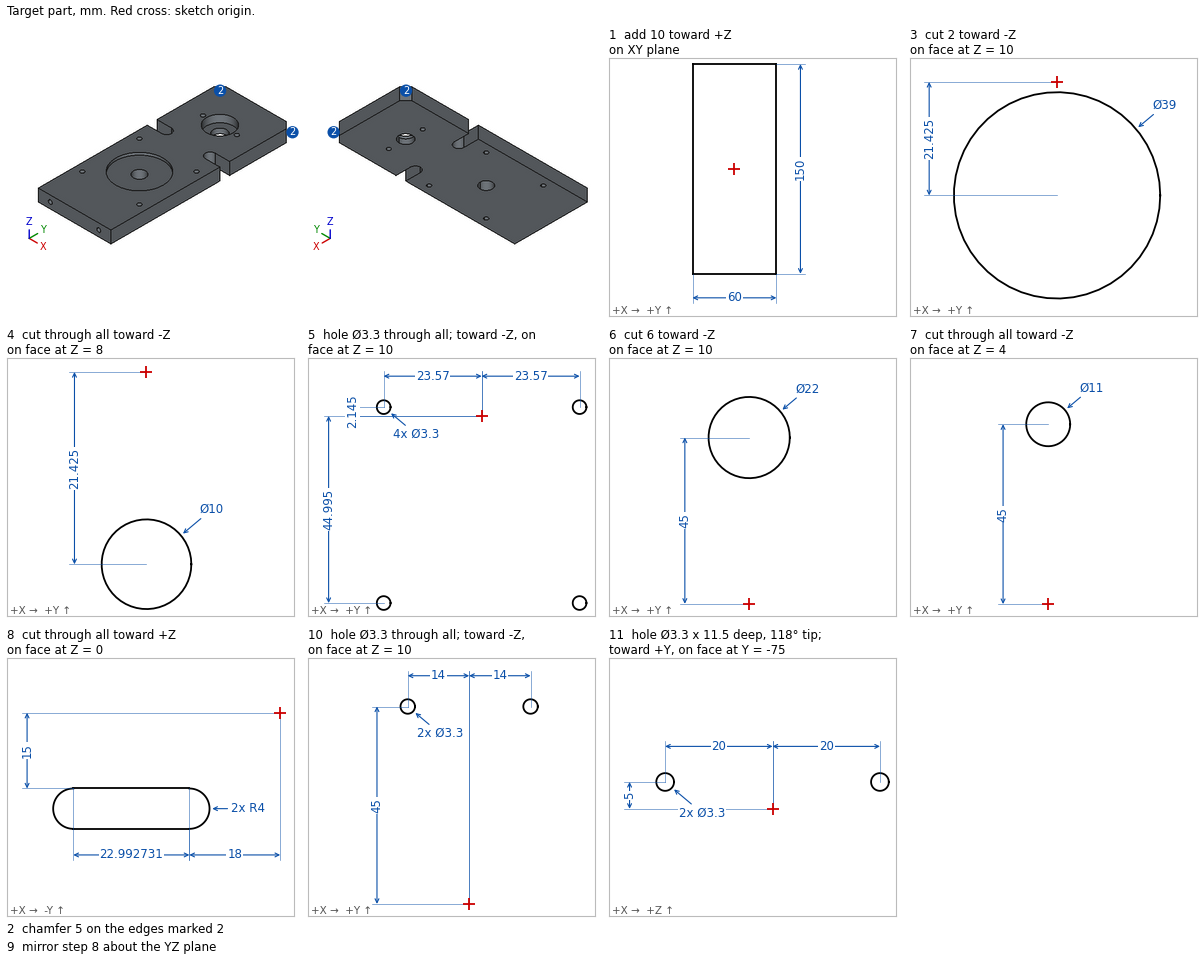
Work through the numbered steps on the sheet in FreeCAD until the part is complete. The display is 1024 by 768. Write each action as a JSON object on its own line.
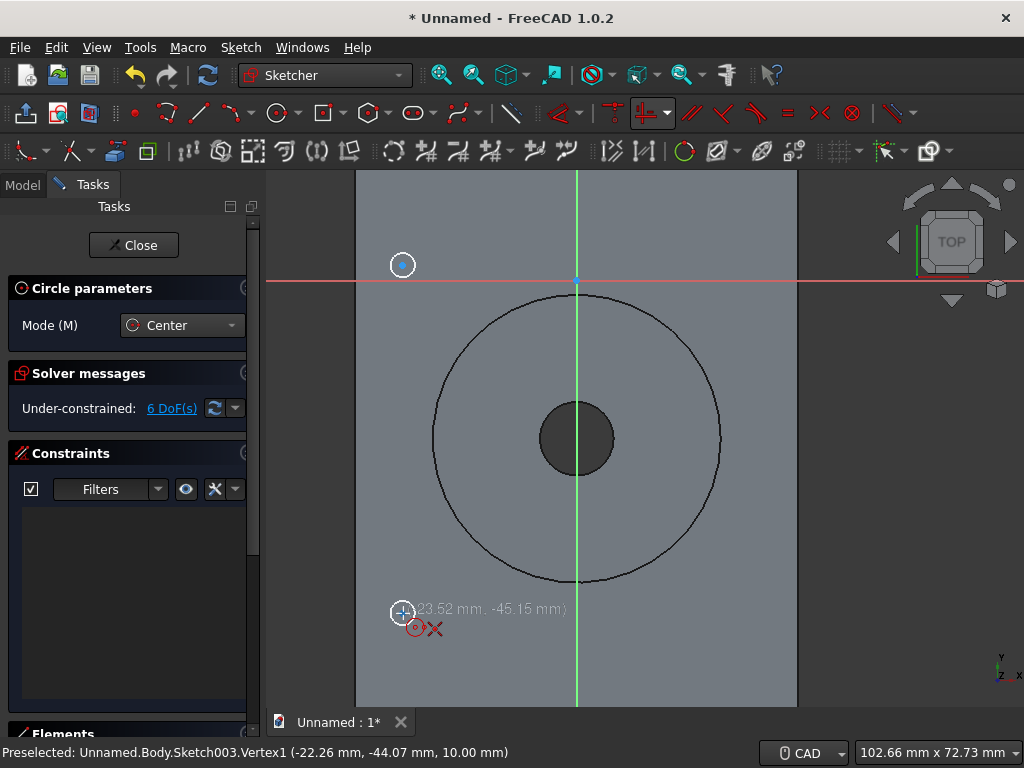
{"action": "scroll", "coordinate": [751, 265], "scroll_direction": "up", "scroll_amount": 4}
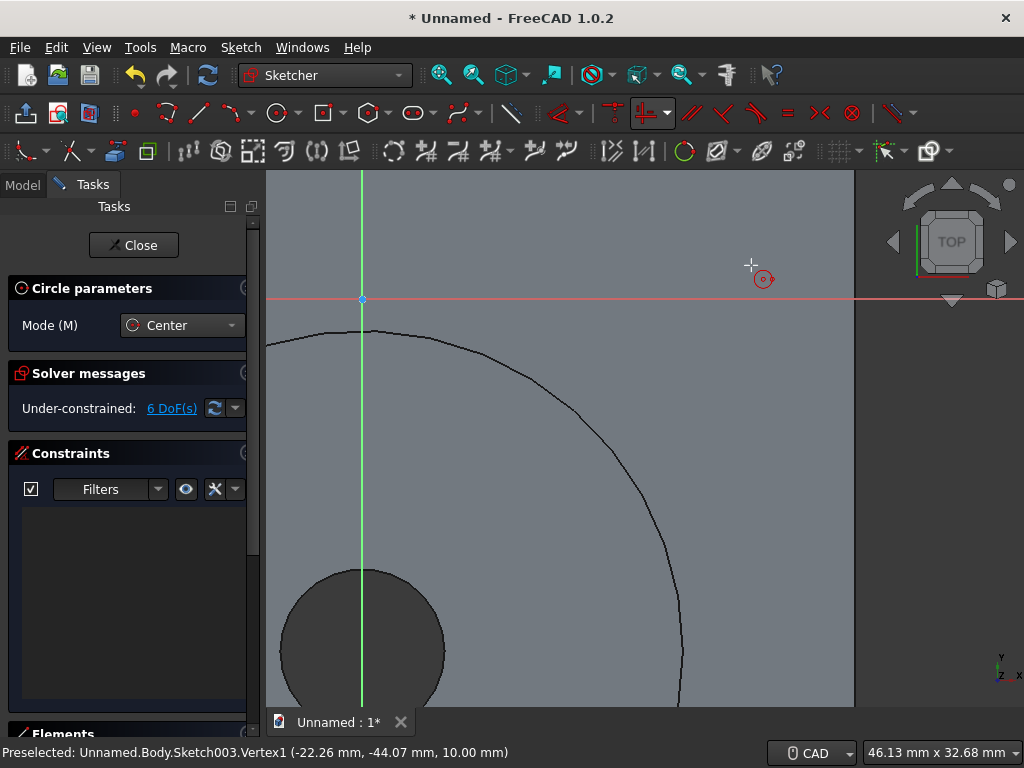
{"action": "left_click", "coordinate": [750, 264]}
{"action": "left_click", "coordinate": [769, 245]}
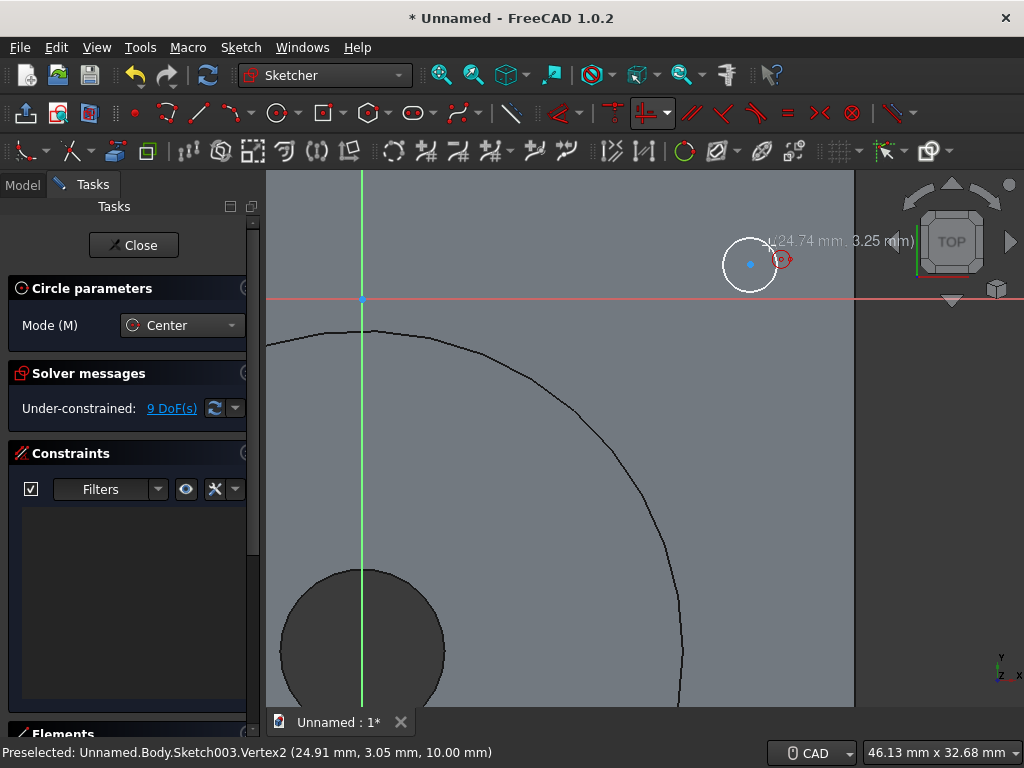
{"action": "scroll", "coordinate": [751, 265], "scroll_direction": "down", "scroll_amount": 4}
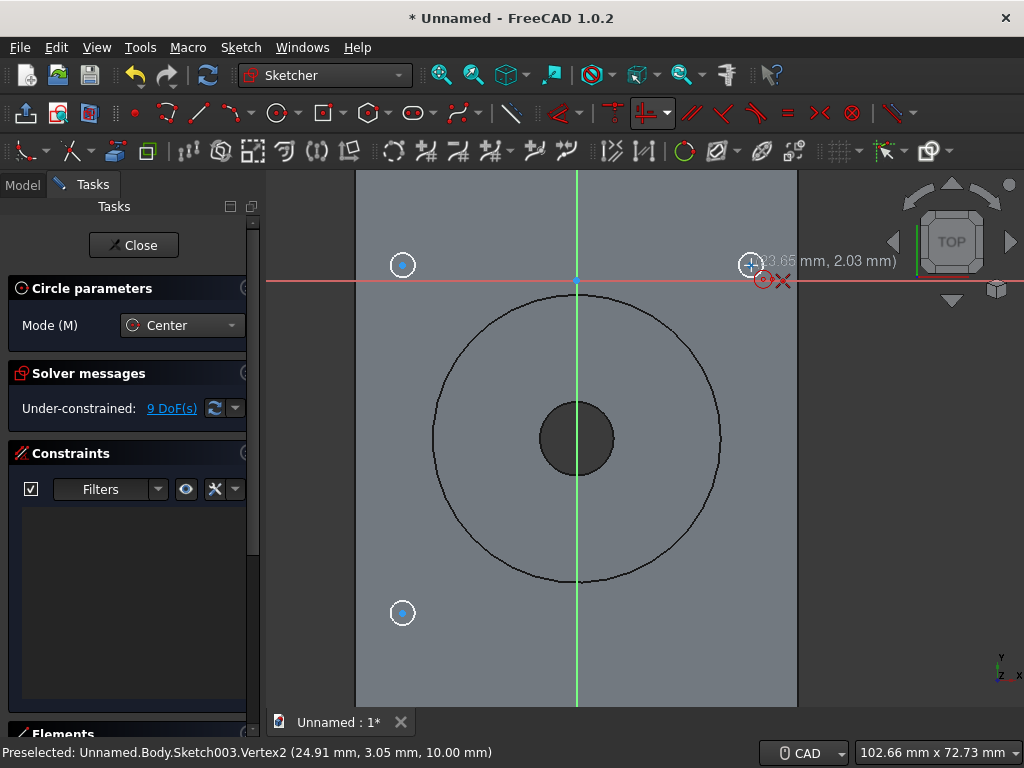
{"action": "scroll", "coordinate": [751, 613], "scroll_direction": "up", "scroll_amount": 4}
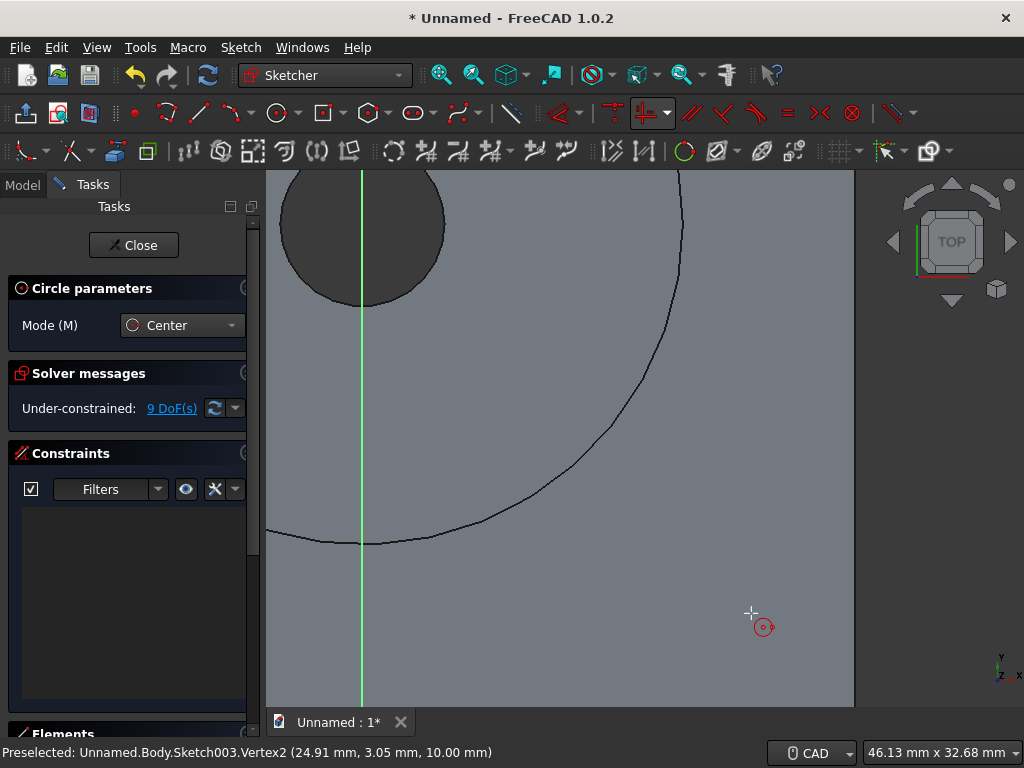
{"action": "left_click", "coordinate": [750, 611]}
{"action": "left_click", "coordinate": [769, 592]}
{"action": "key", "text": "Escape"}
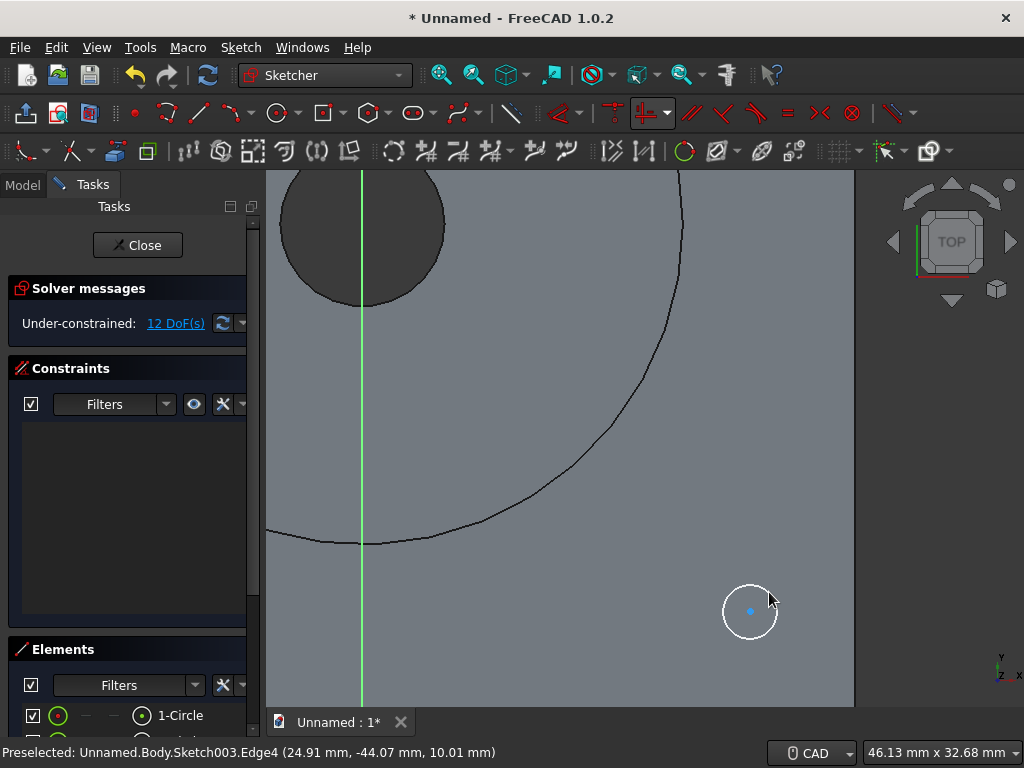
{"action": "scroll", "coordinate": [751, 613], "scroll_direction": "down", "scroll_amount": 4}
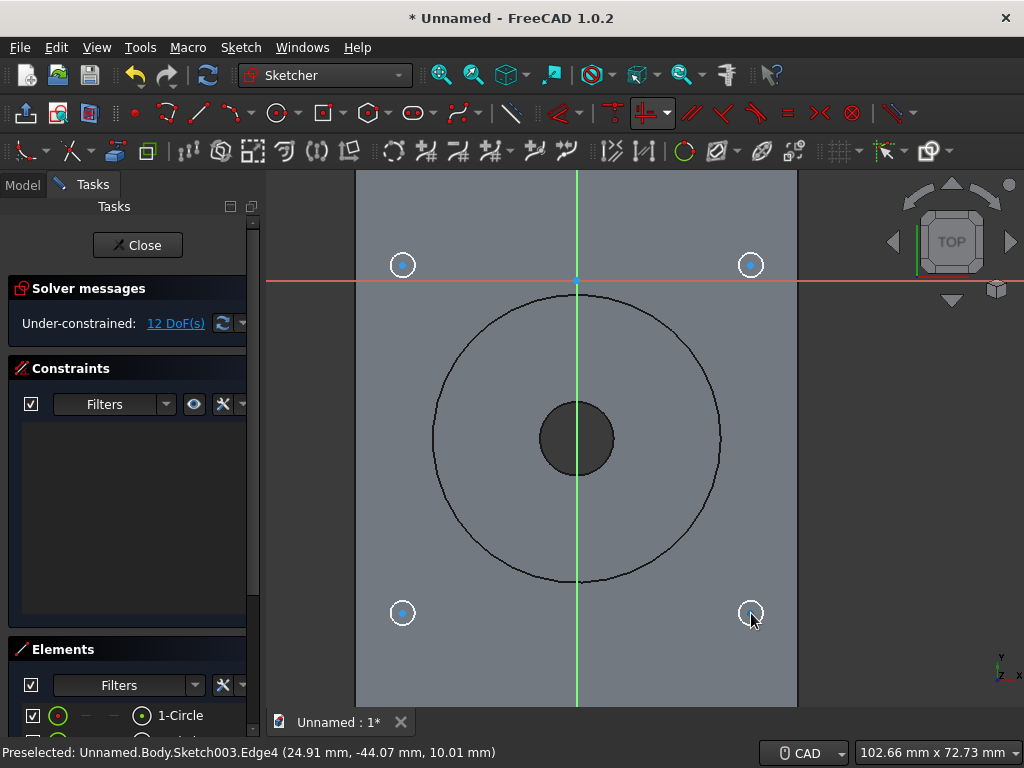
{"action": "left_click", "coordinate": [411, 257]}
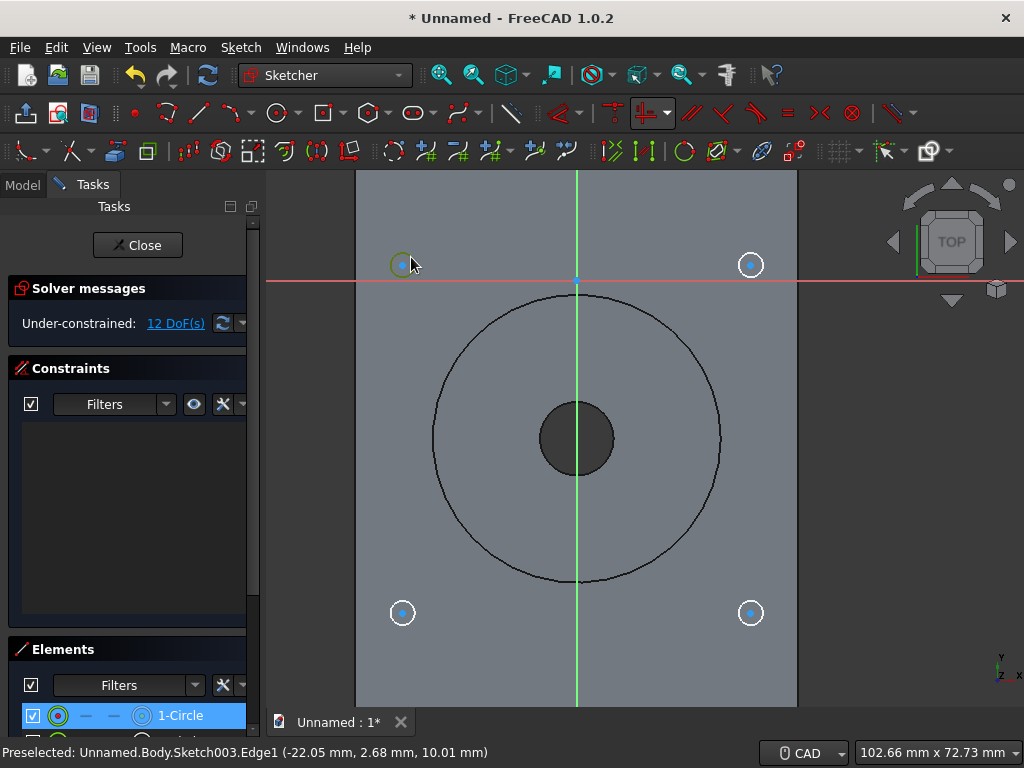
{"action": "left_click", "coordinate": [411, 604]}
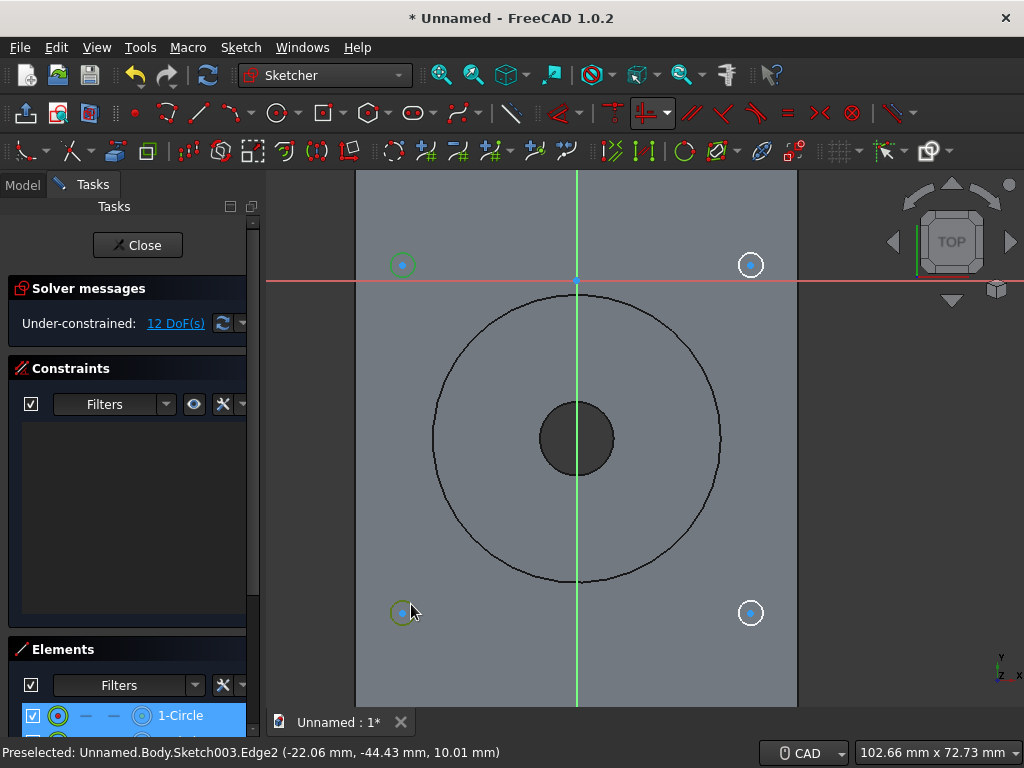
{"action": "left_click", "coordinate": [759, 257]}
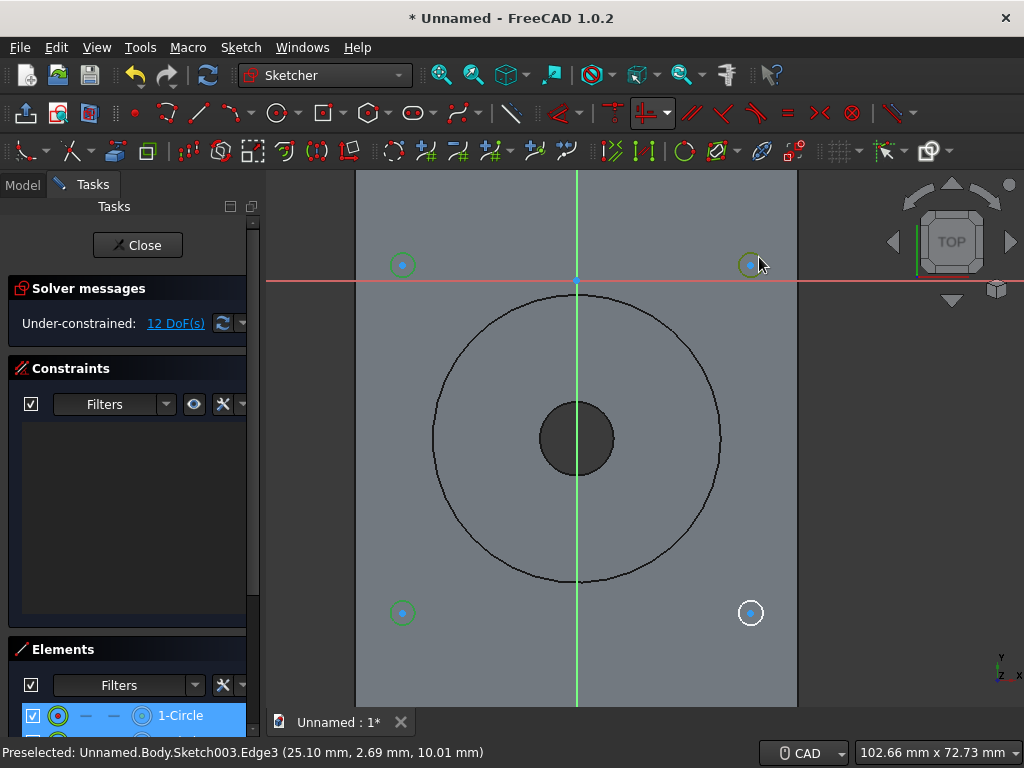
{"action": "left_click", "coordinate": [759, 604]}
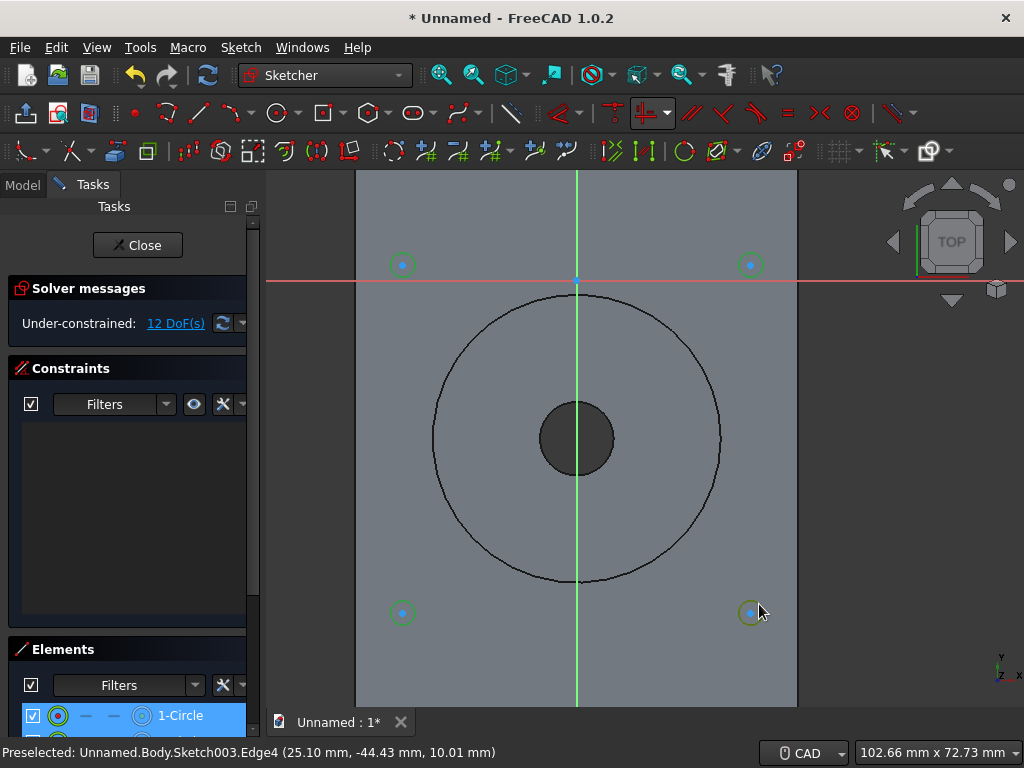
{"action": "left_click", "coordinate": [788, 114]}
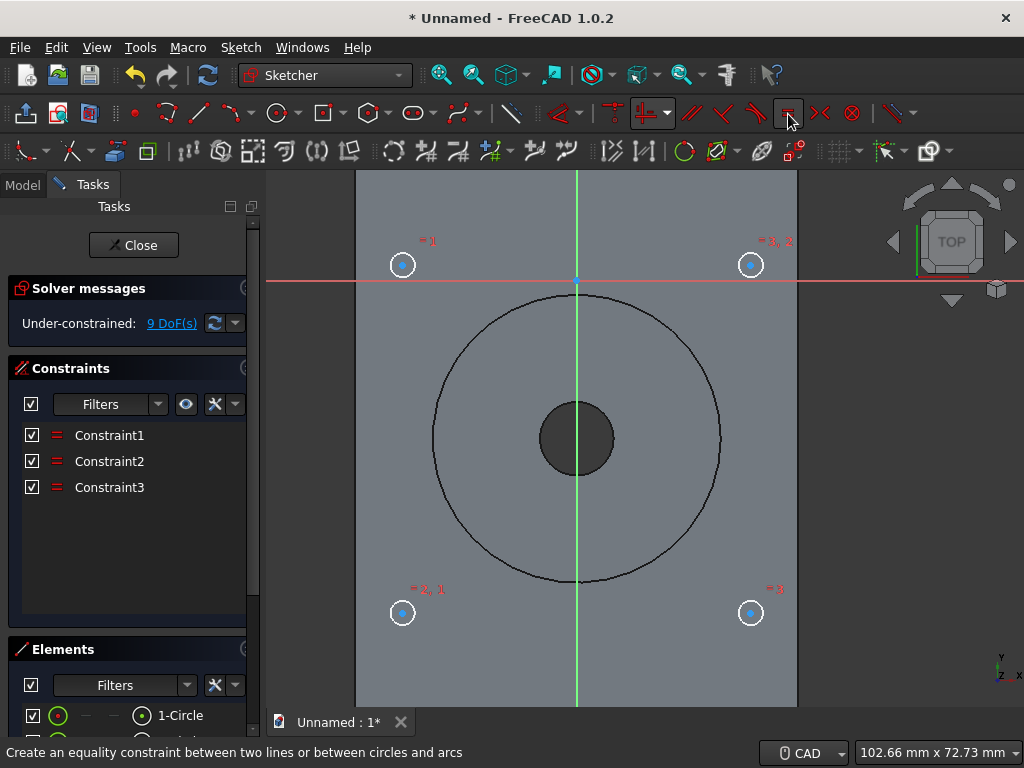
{"action": "left_click", "coordinate": [403, 265]}